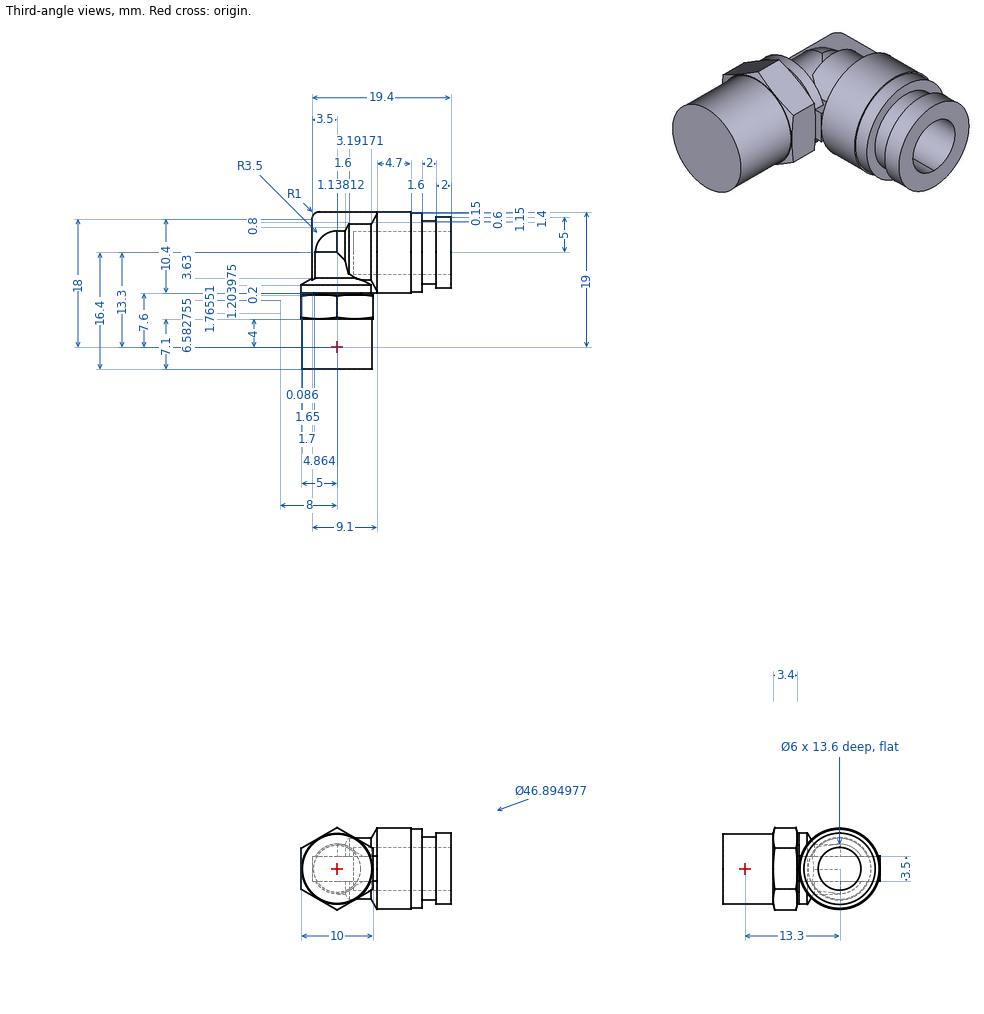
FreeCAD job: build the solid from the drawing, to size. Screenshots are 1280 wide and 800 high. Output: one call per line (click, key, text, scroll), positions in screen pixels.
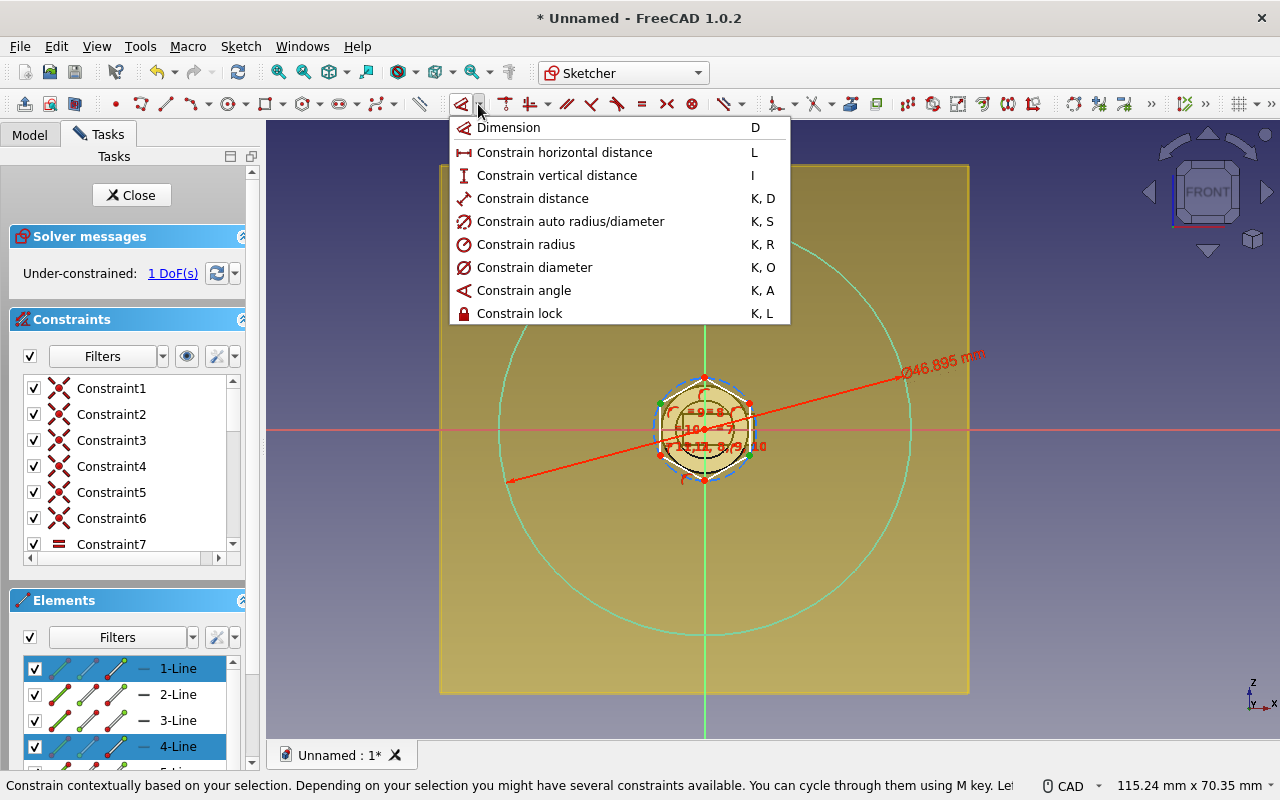
click(620, 152)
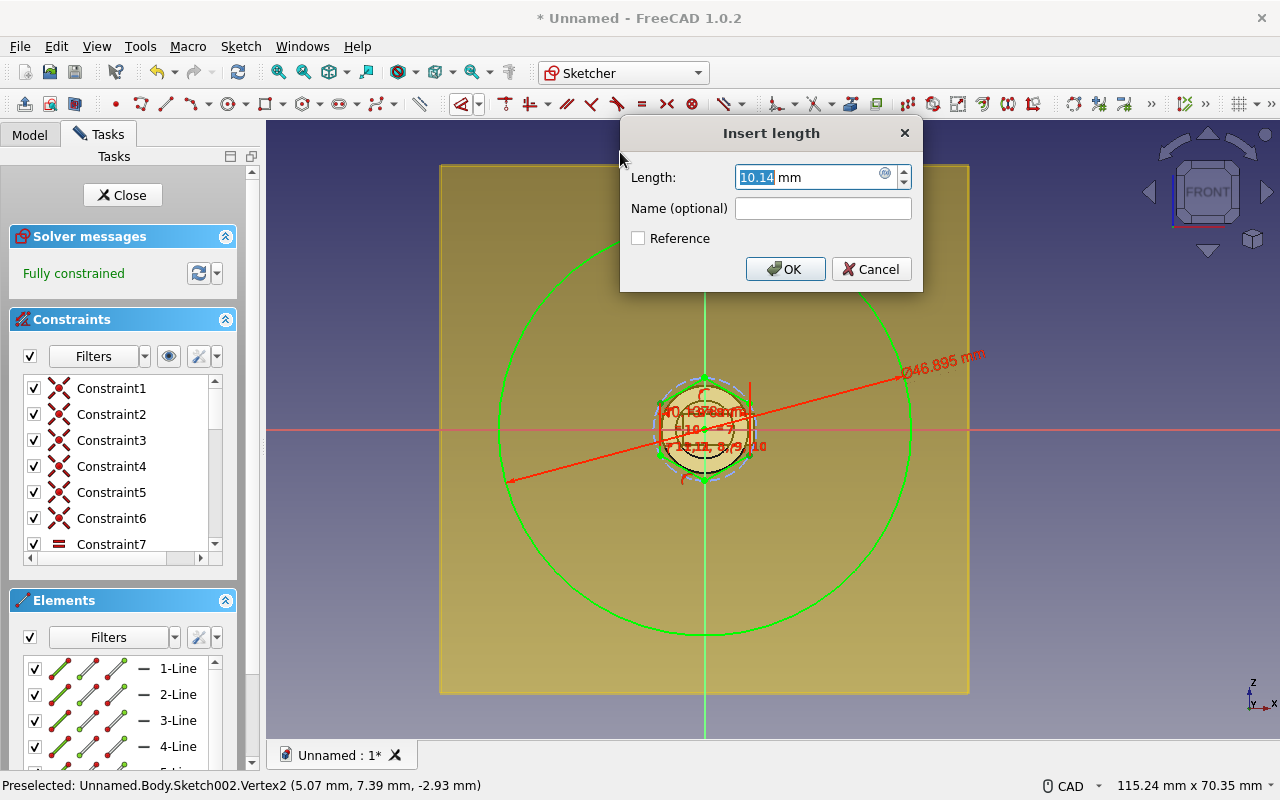
text(10)
key(Return)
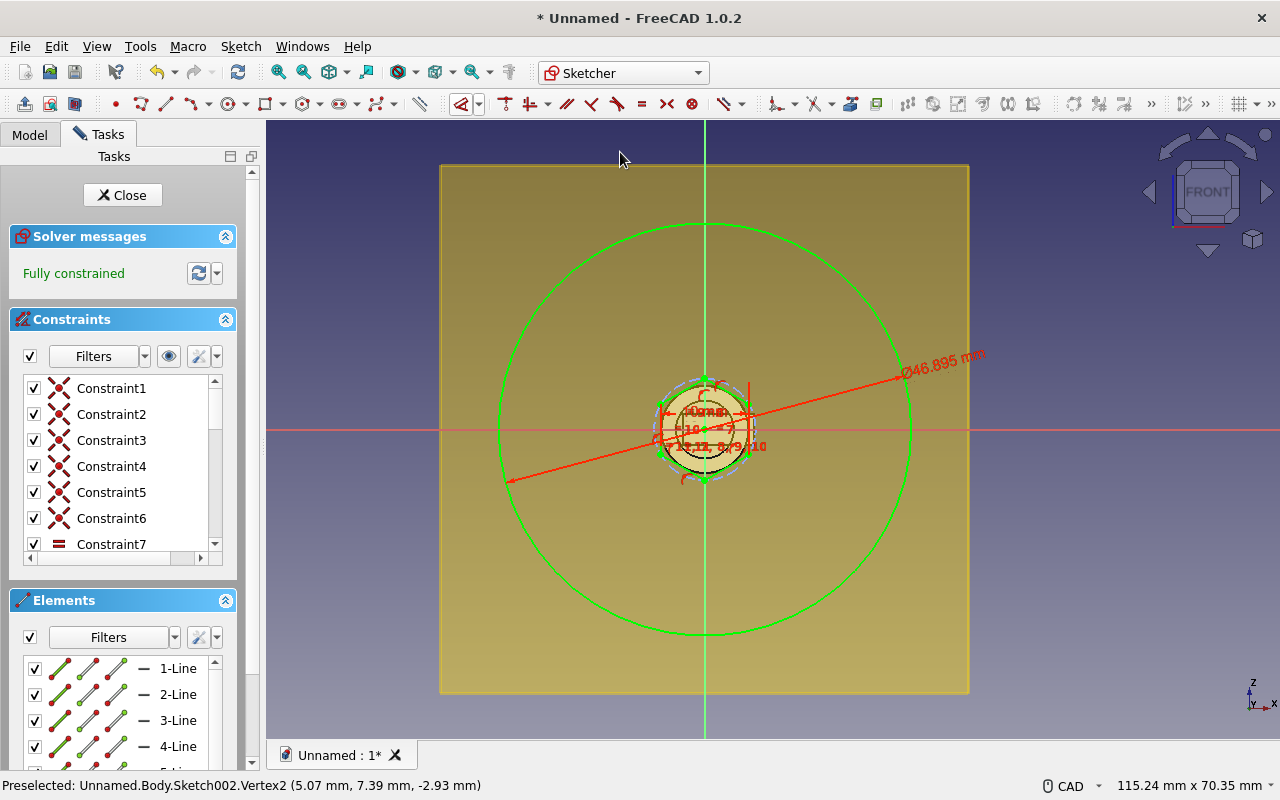
click(123, 195)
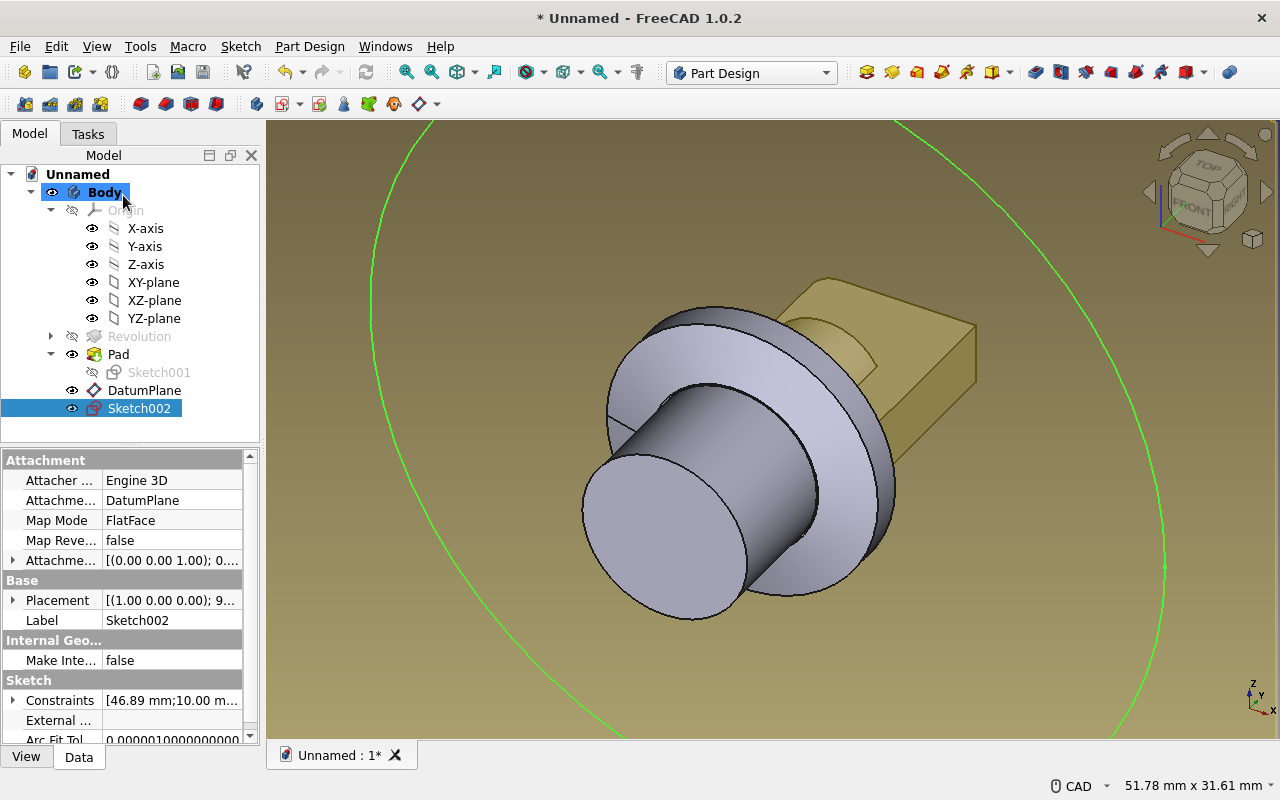
click(1036, 72)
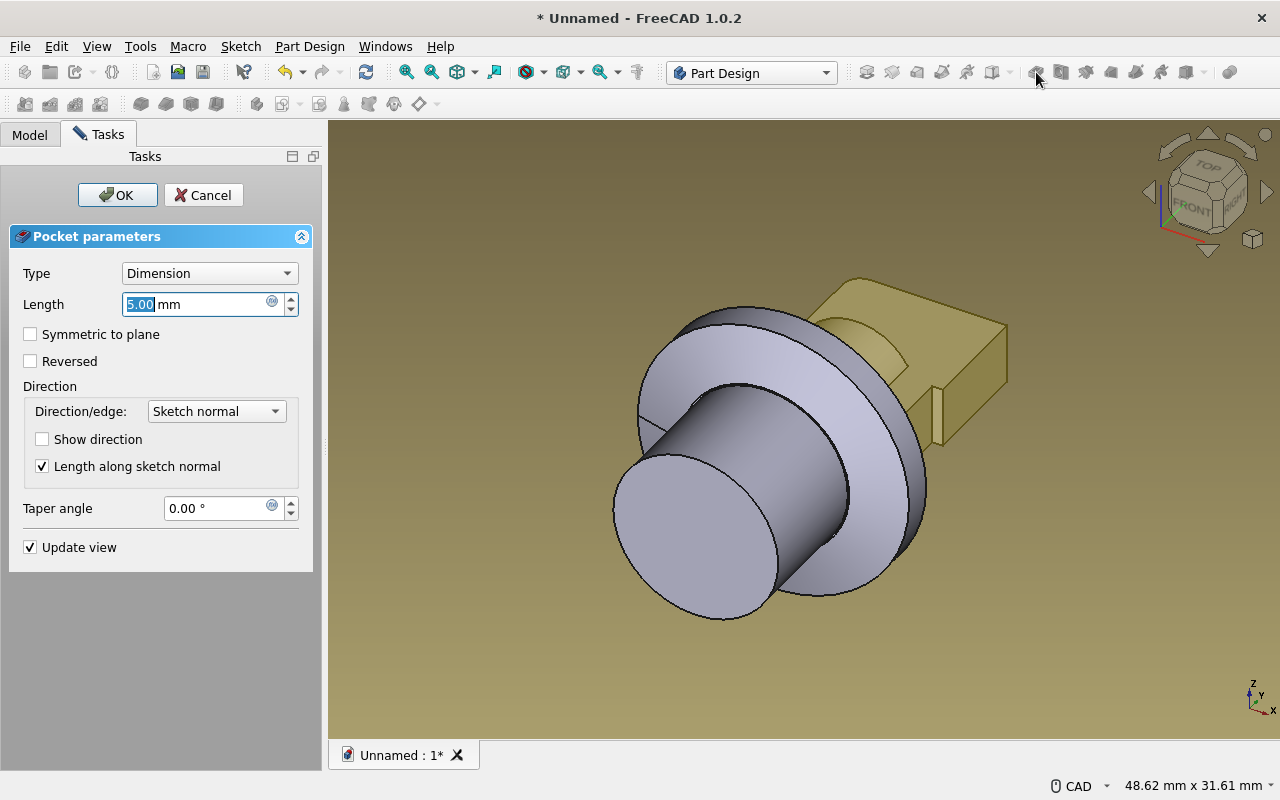
text(3.4)
key(Tab)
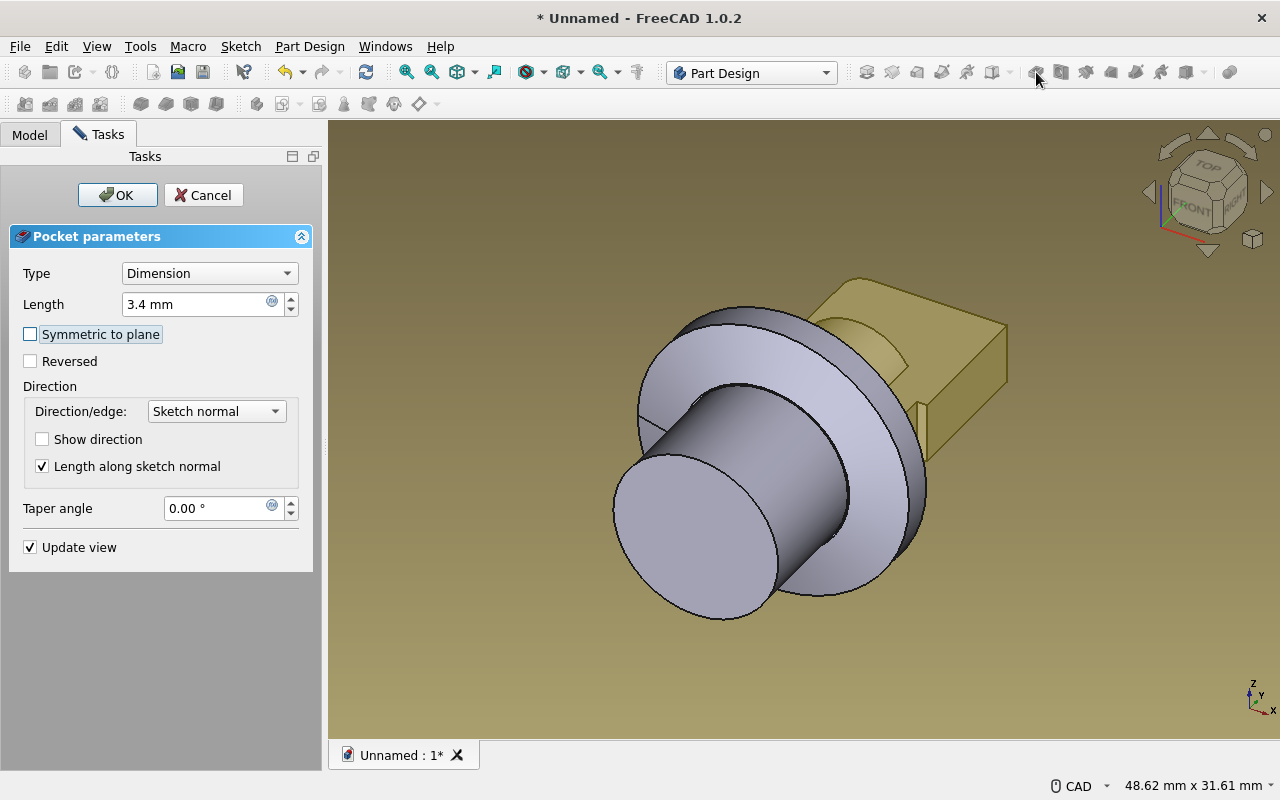
click(31, 361)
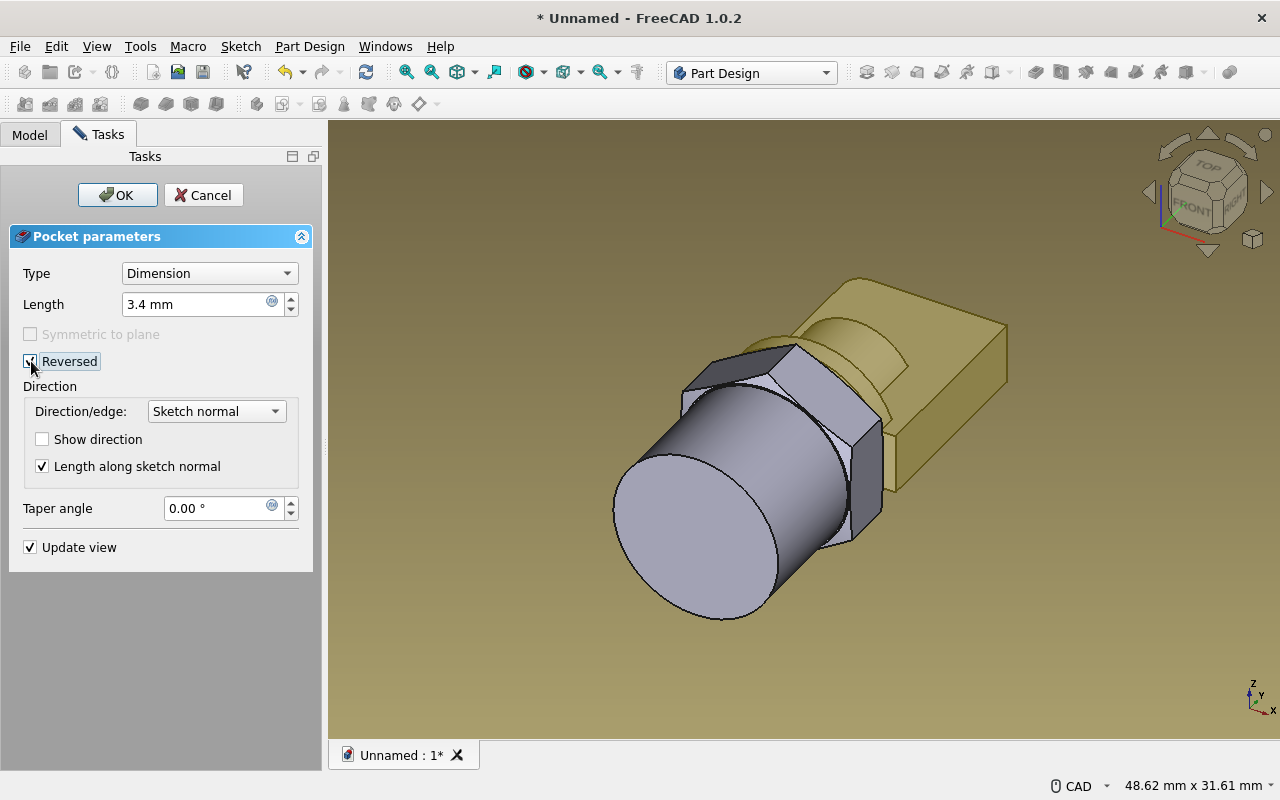
click(118, 195)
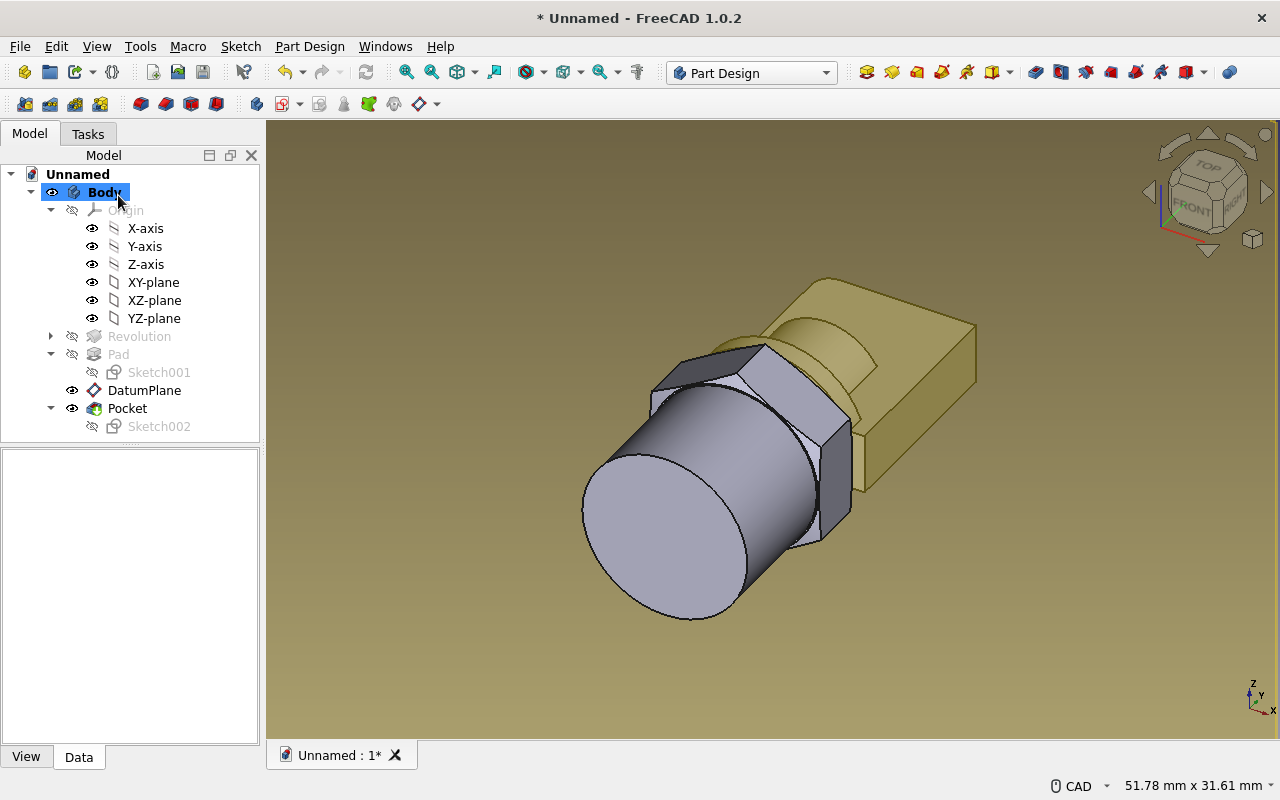
click(117, 390)
key(space)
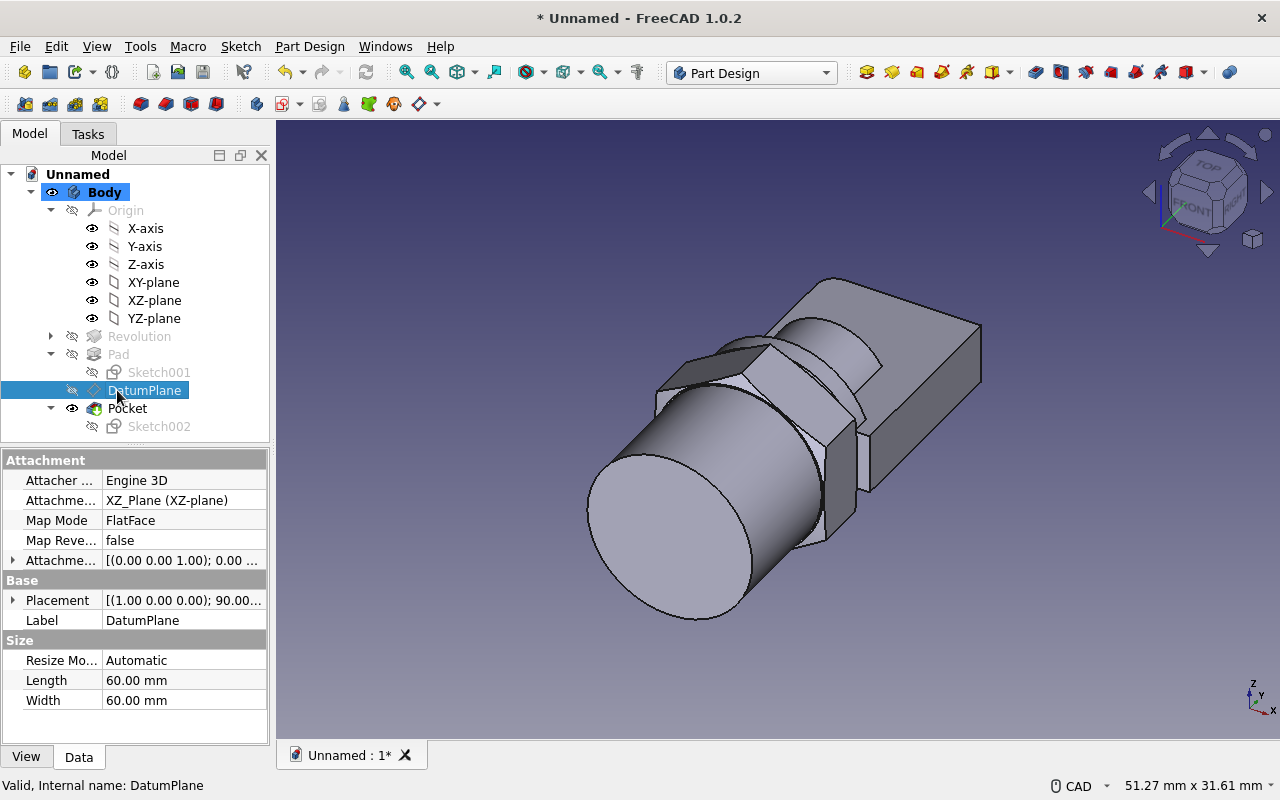
click(316, 699)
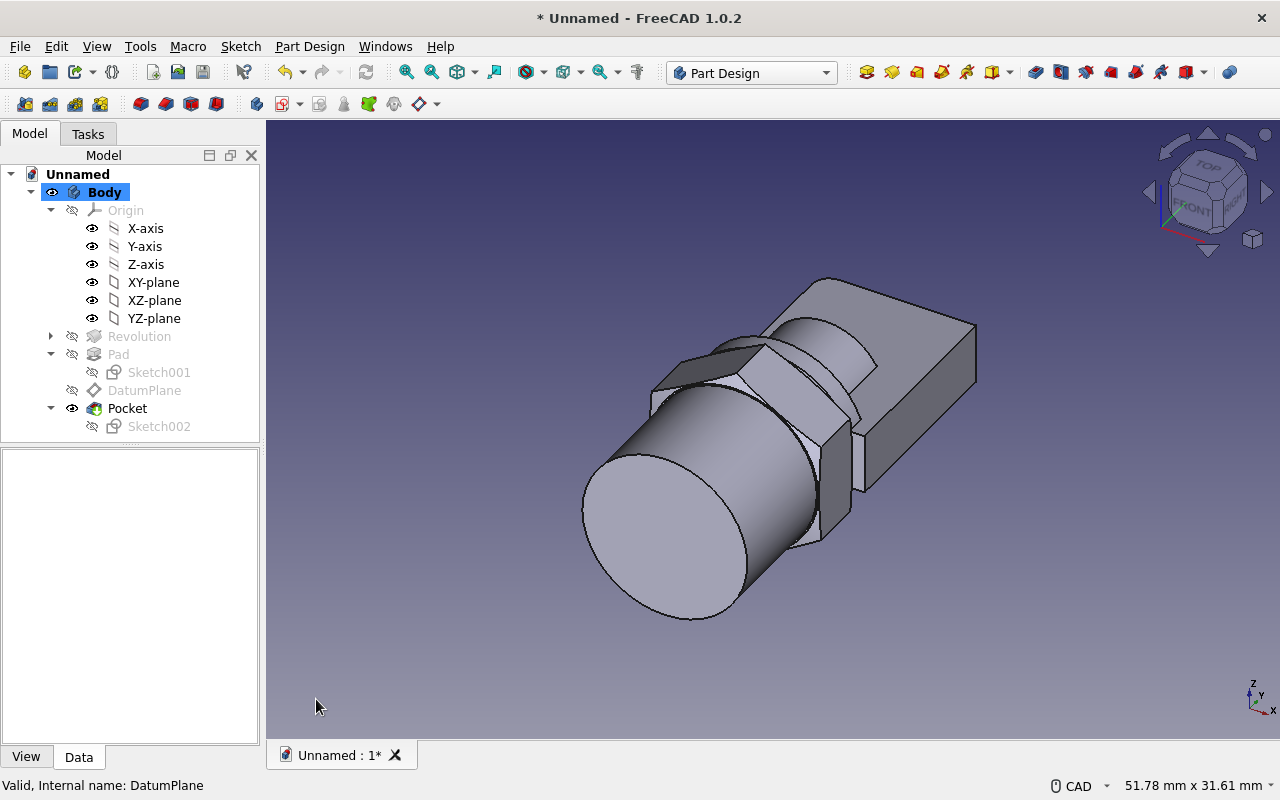
click(282, 104)